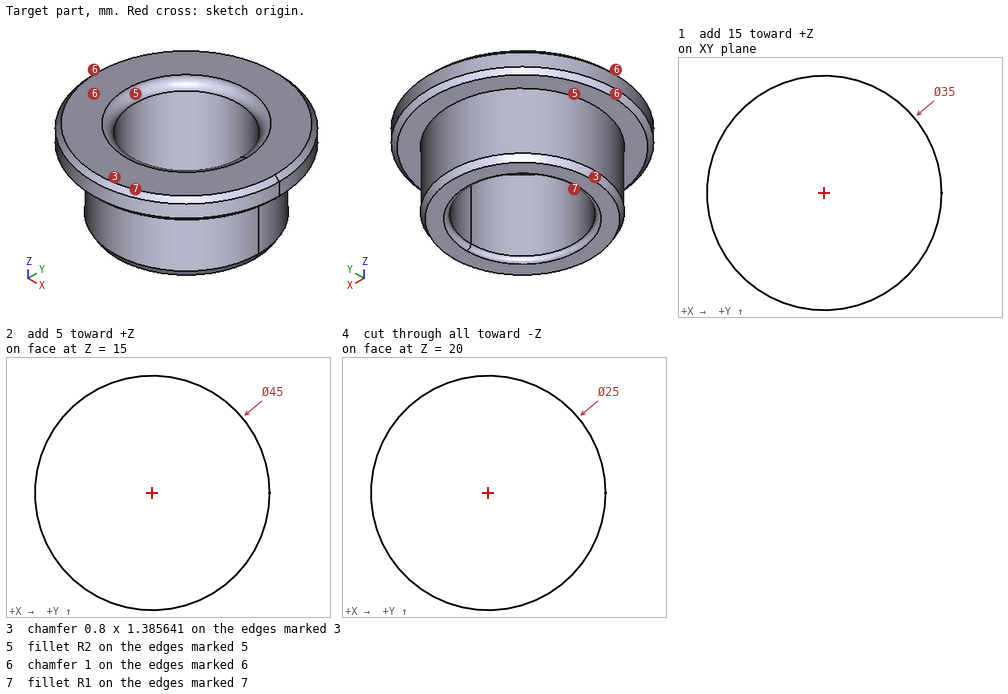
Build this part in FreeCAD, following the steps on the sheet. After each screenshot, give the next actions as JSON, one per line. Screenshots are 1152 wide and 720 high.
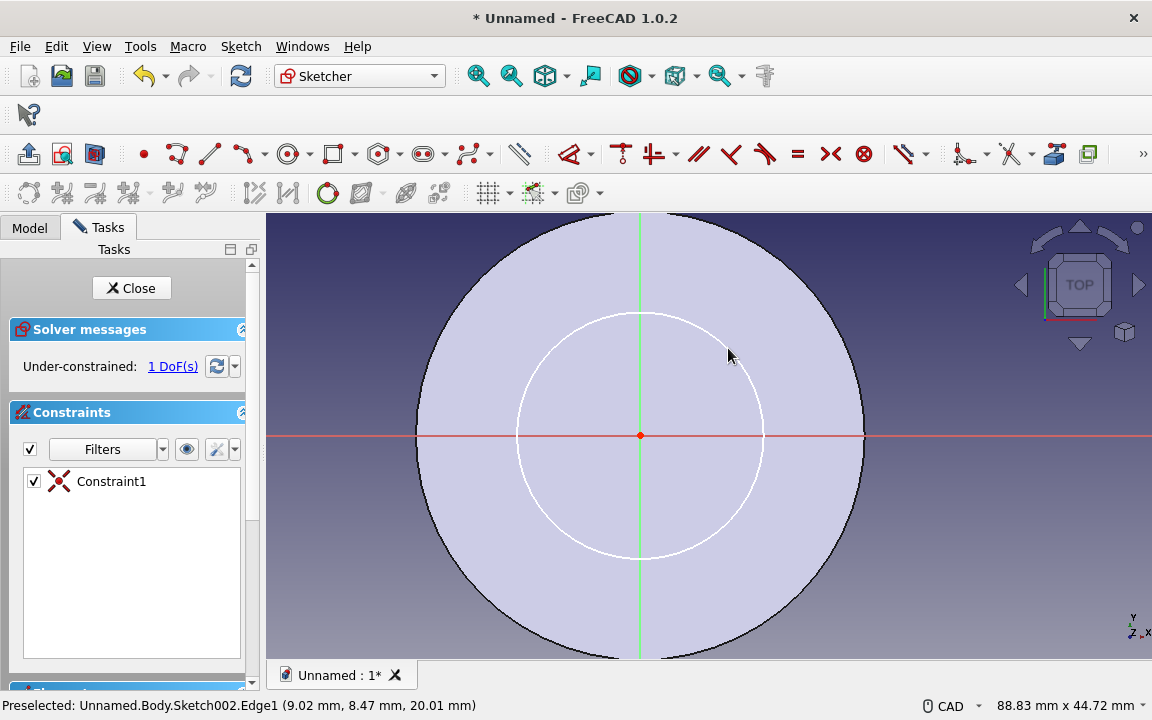
{"action": "left_click", "coordinate": [568, 154]}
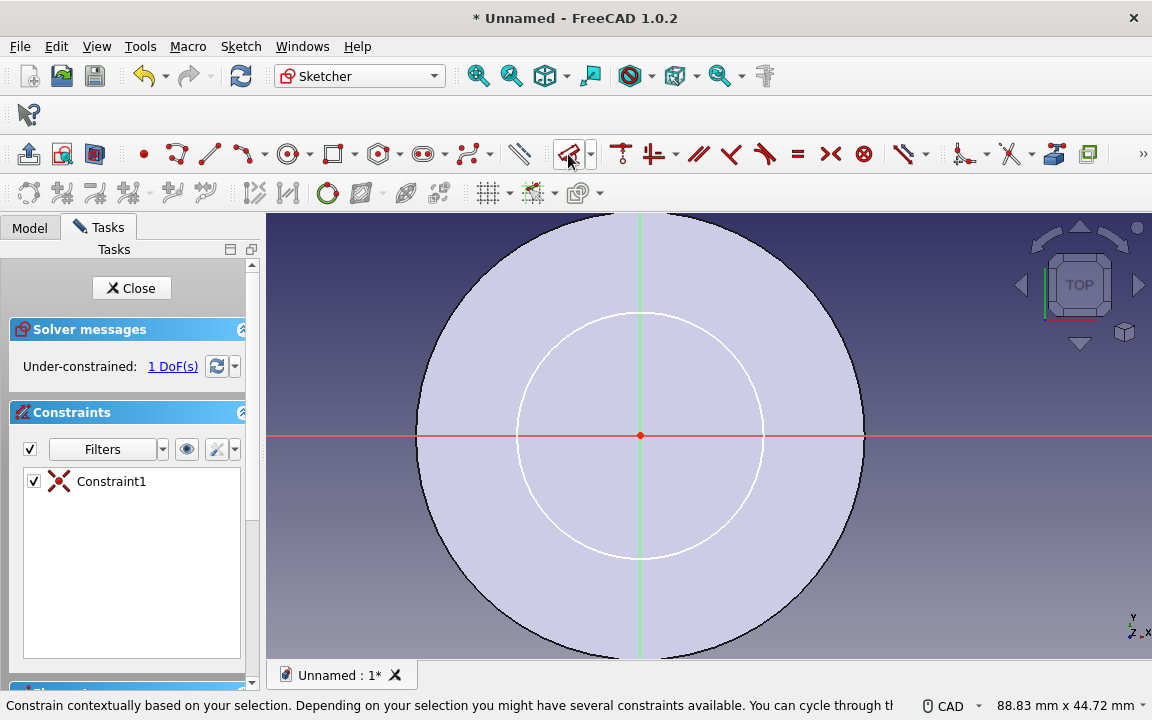
{"action": "left_click", "coordinate": [727, 348]}
{"action": "left_click", "coordinate": [749, 325]}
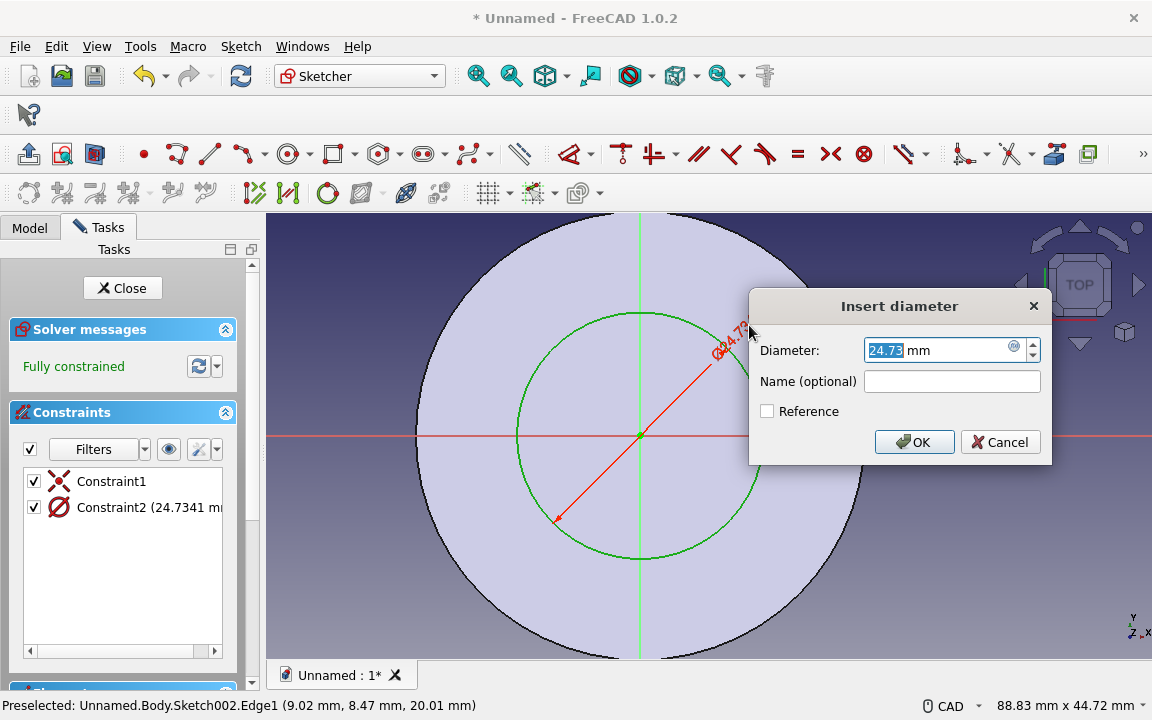
{"action": "type", "text": "25"}
{"action": "key", "text": "Return"}
{"action": "key", "text": "Escape"}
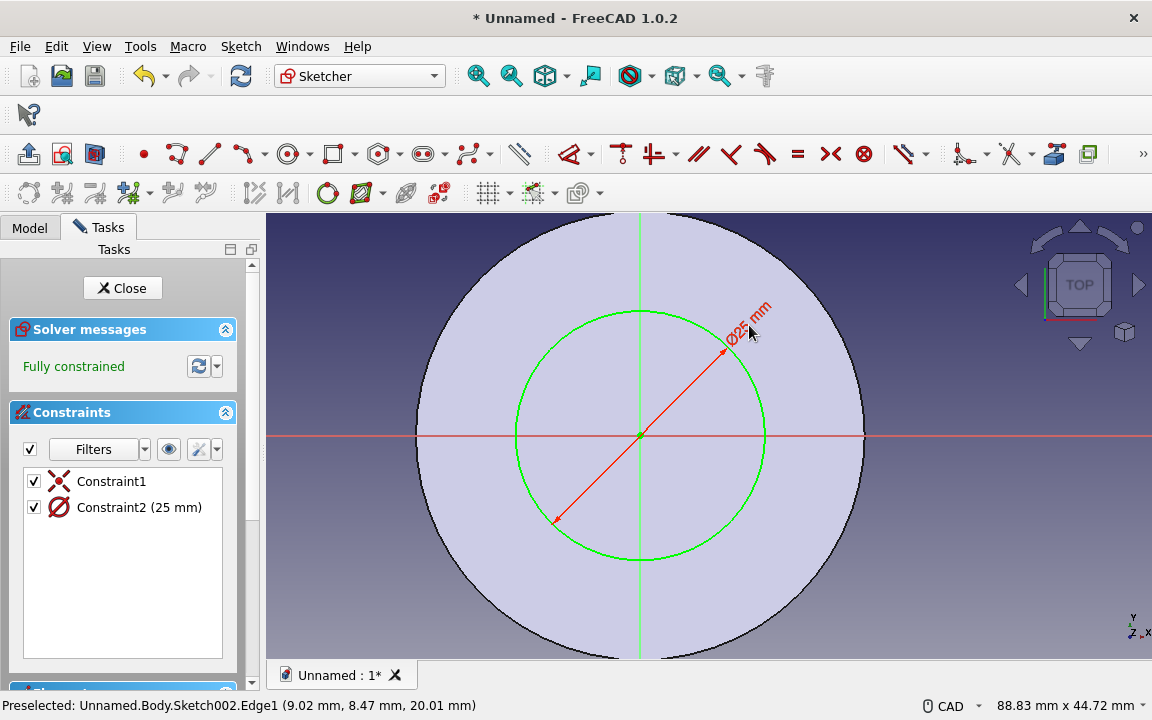
{"action": "left_click", "coordinate": [123, 288]}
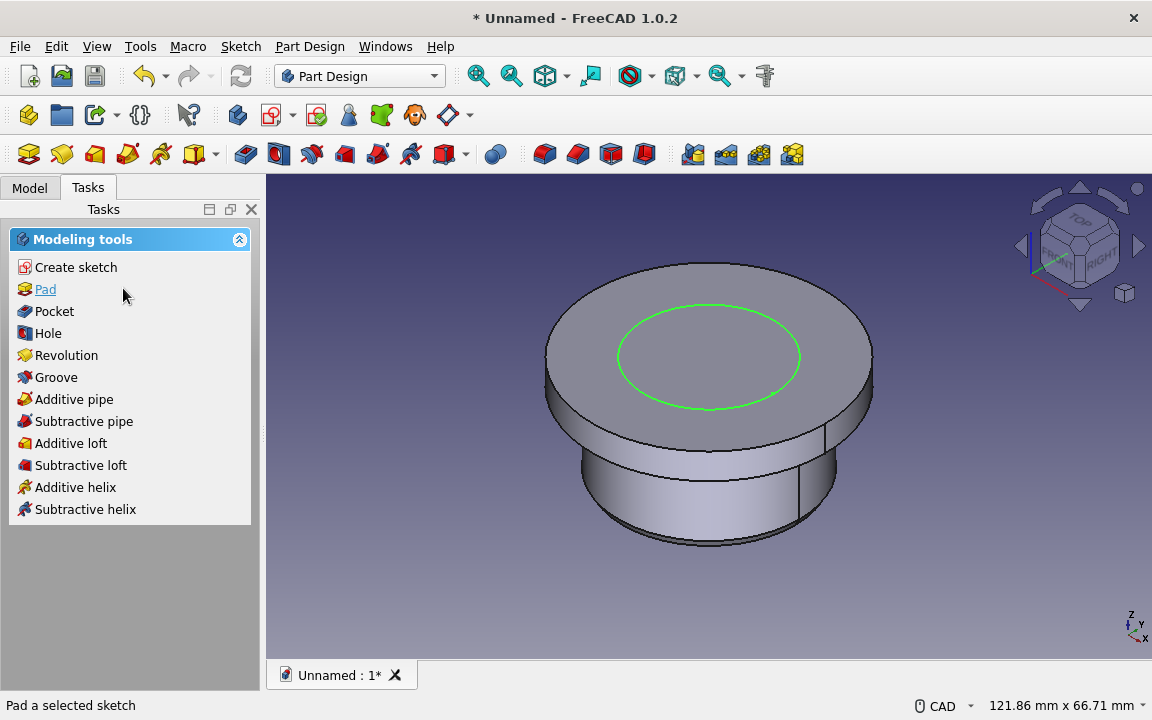
{"action": "left_click", "coordinate": [246, 154]}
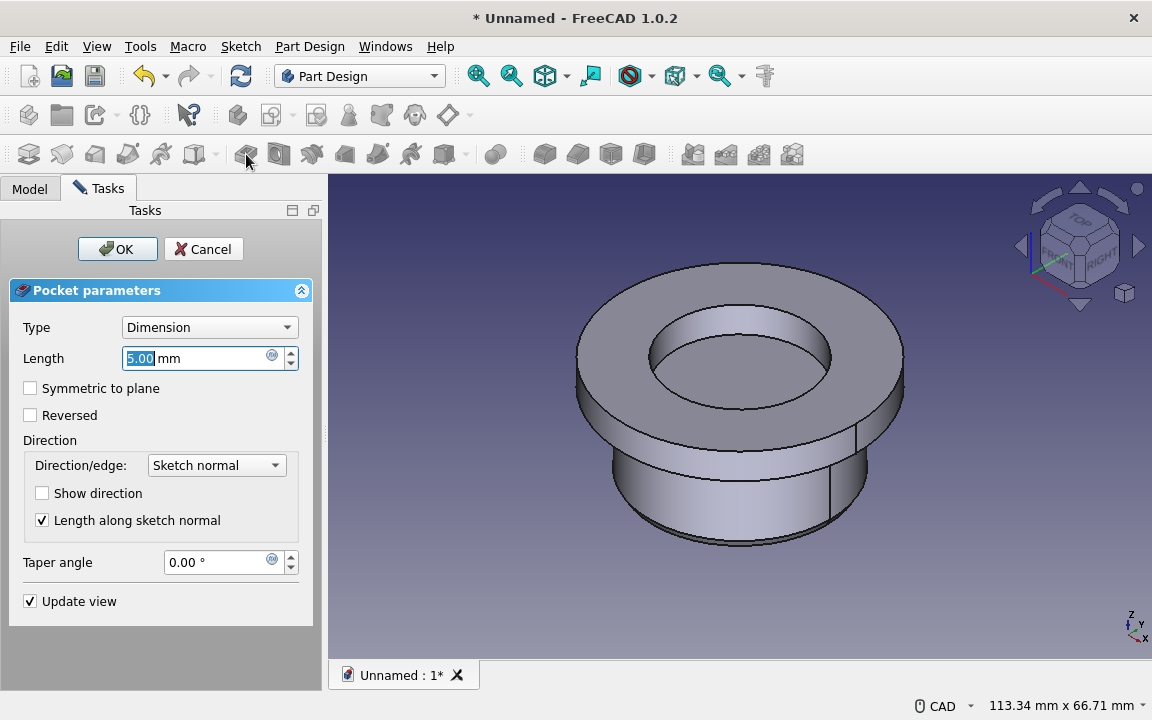
{"action": "left_click", "coordinate": [210, 328]}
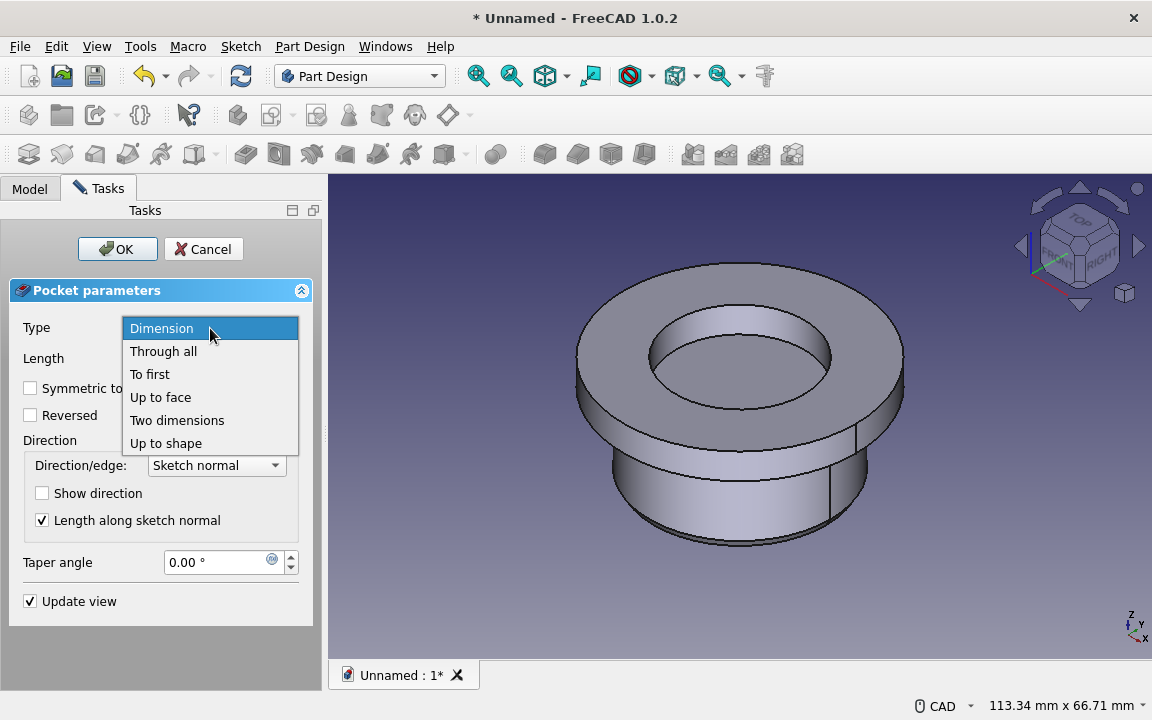
{"action": "left_click", "coordinate": [208, 352]}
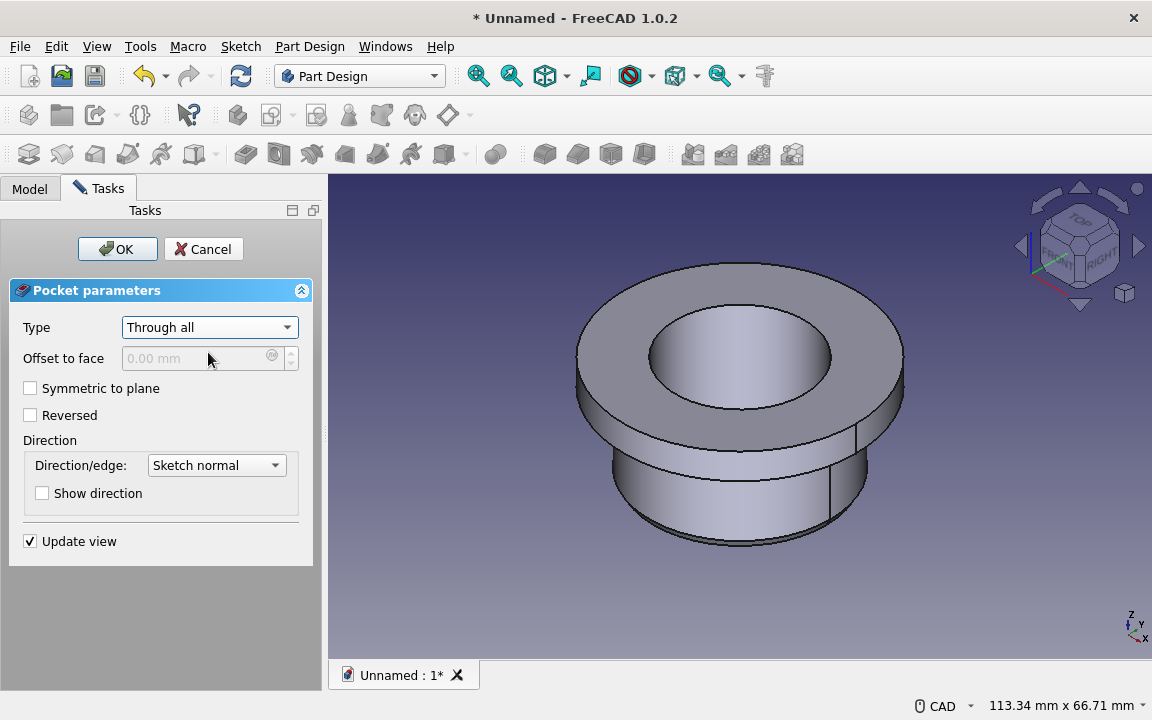
{"action": "left_click", "coordinate": [118, 249]}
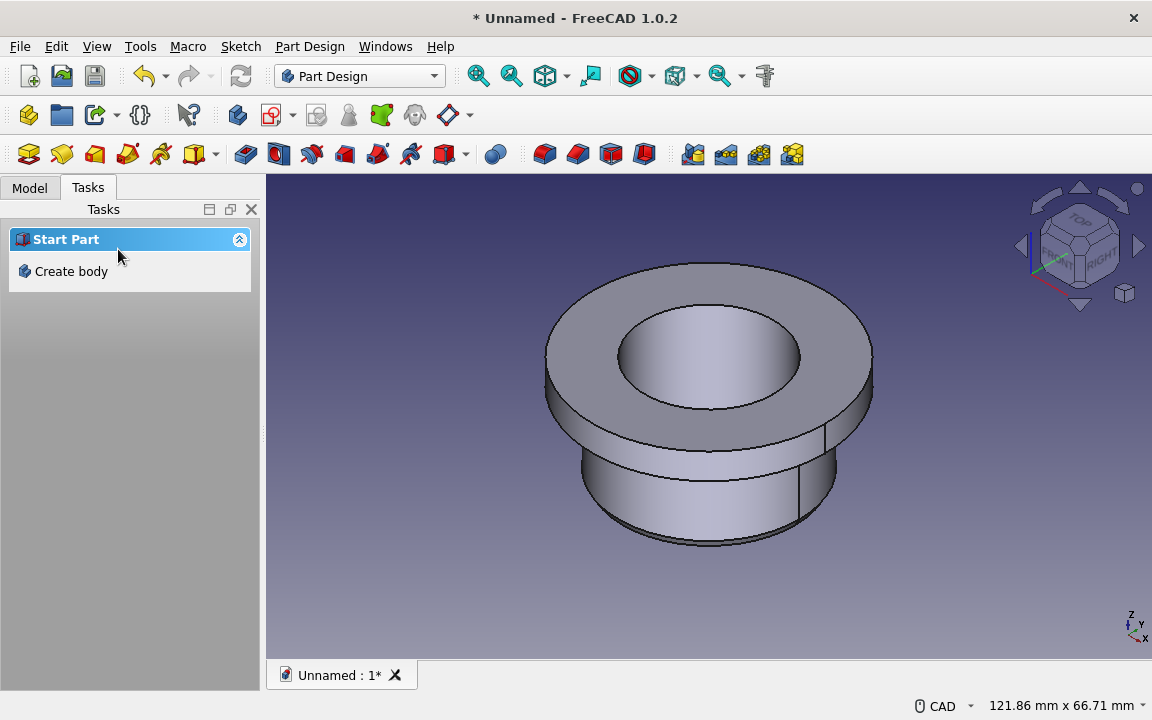
{"action": "left_click", "coordinate": [645, 319]}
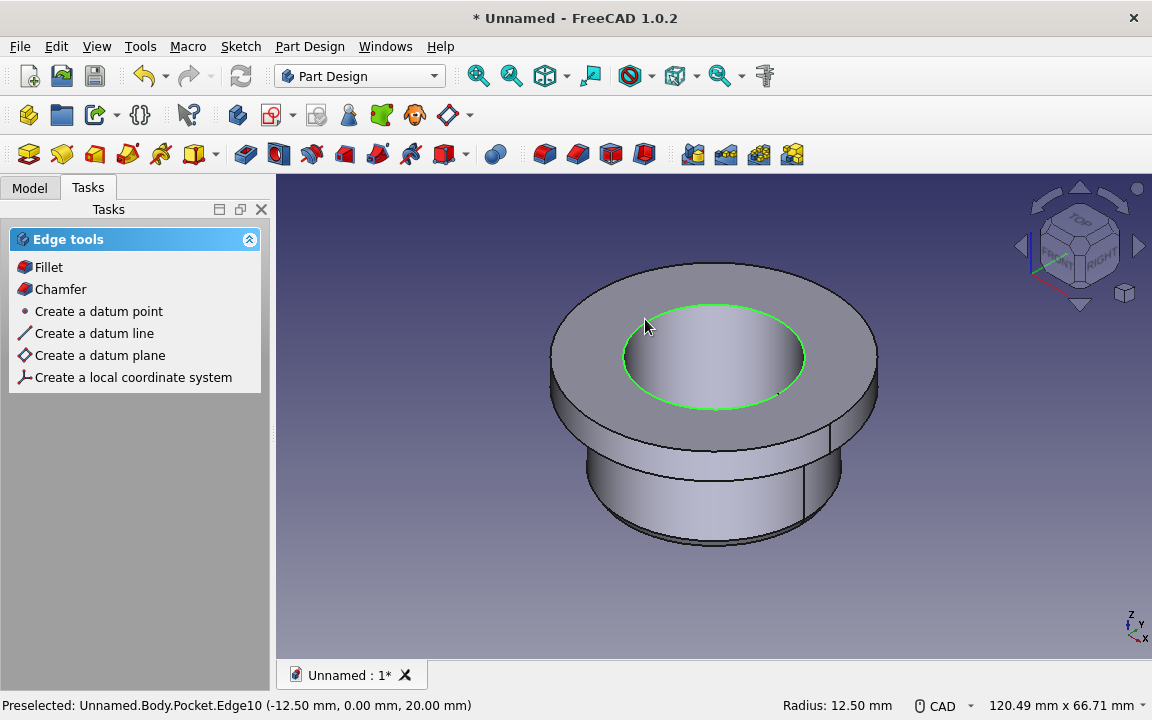
{"action": "left_click", "coordinate": [545, 154]}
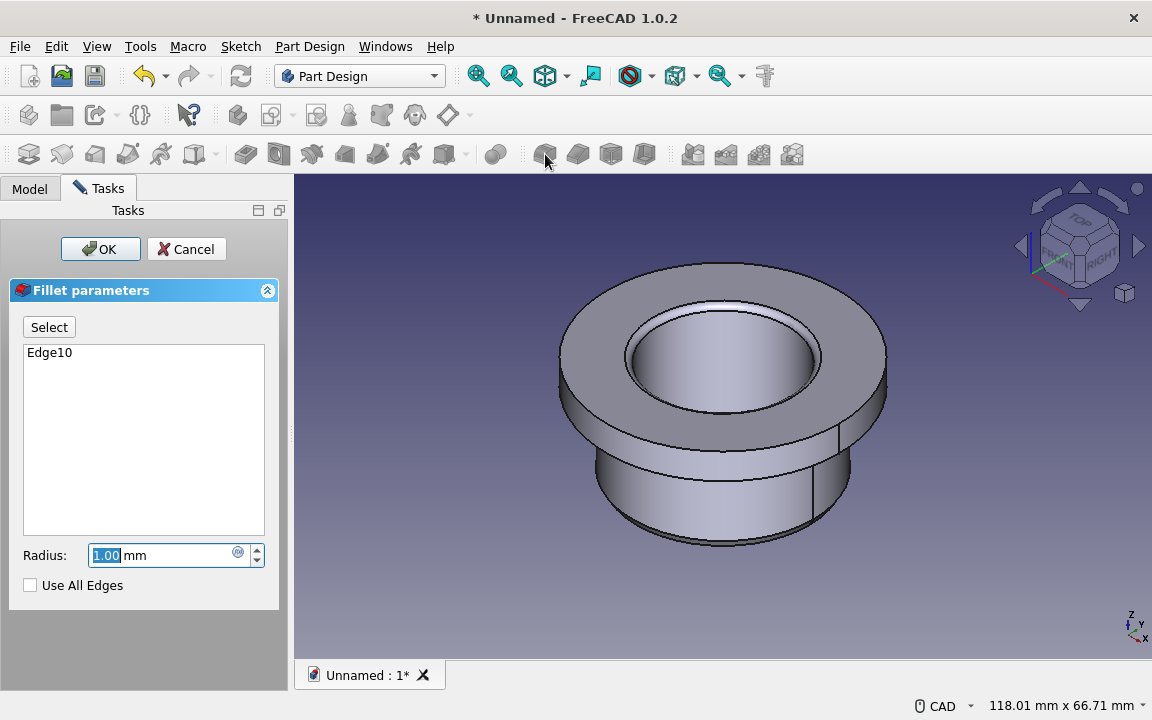
{"action": "type", "text": "2"}
{"action": "key", "text": "Tab"}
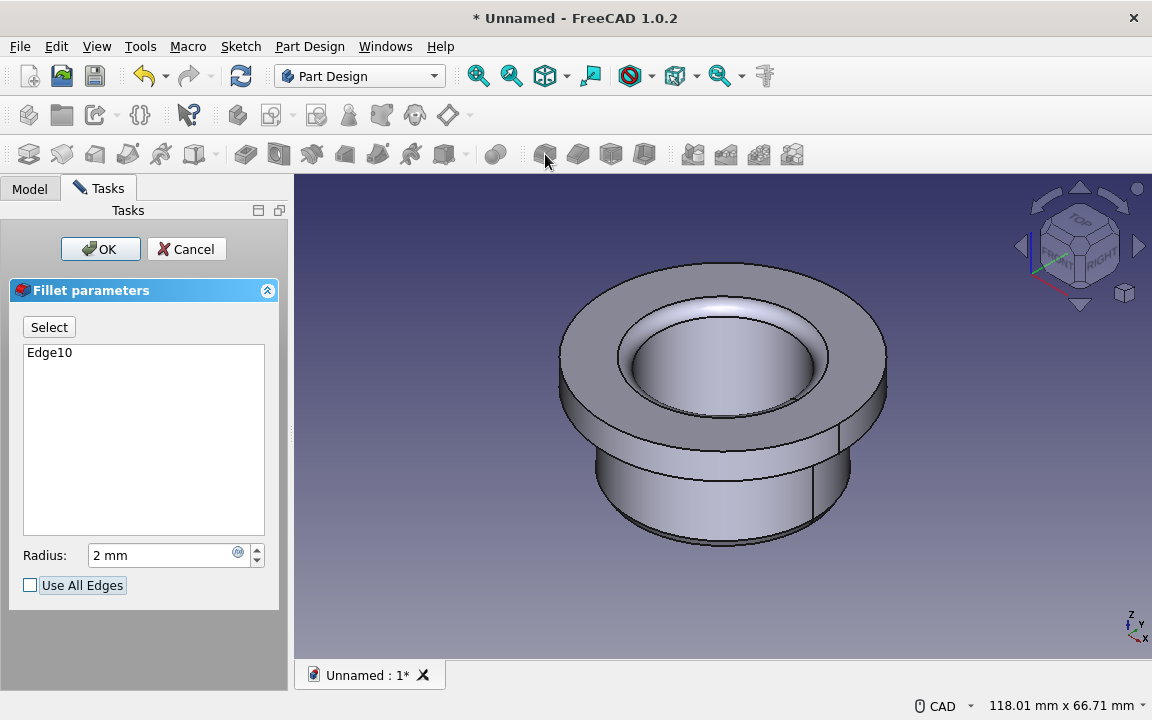
{"action": "left_click", "coordinate": [101, 249]}